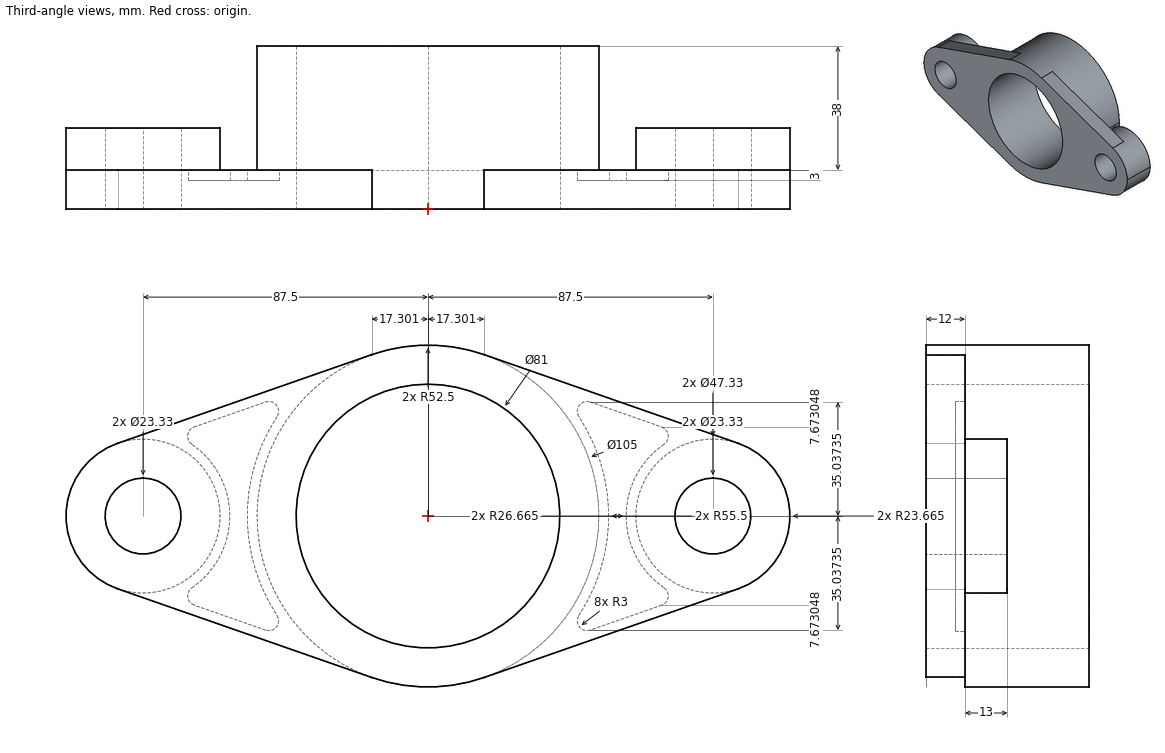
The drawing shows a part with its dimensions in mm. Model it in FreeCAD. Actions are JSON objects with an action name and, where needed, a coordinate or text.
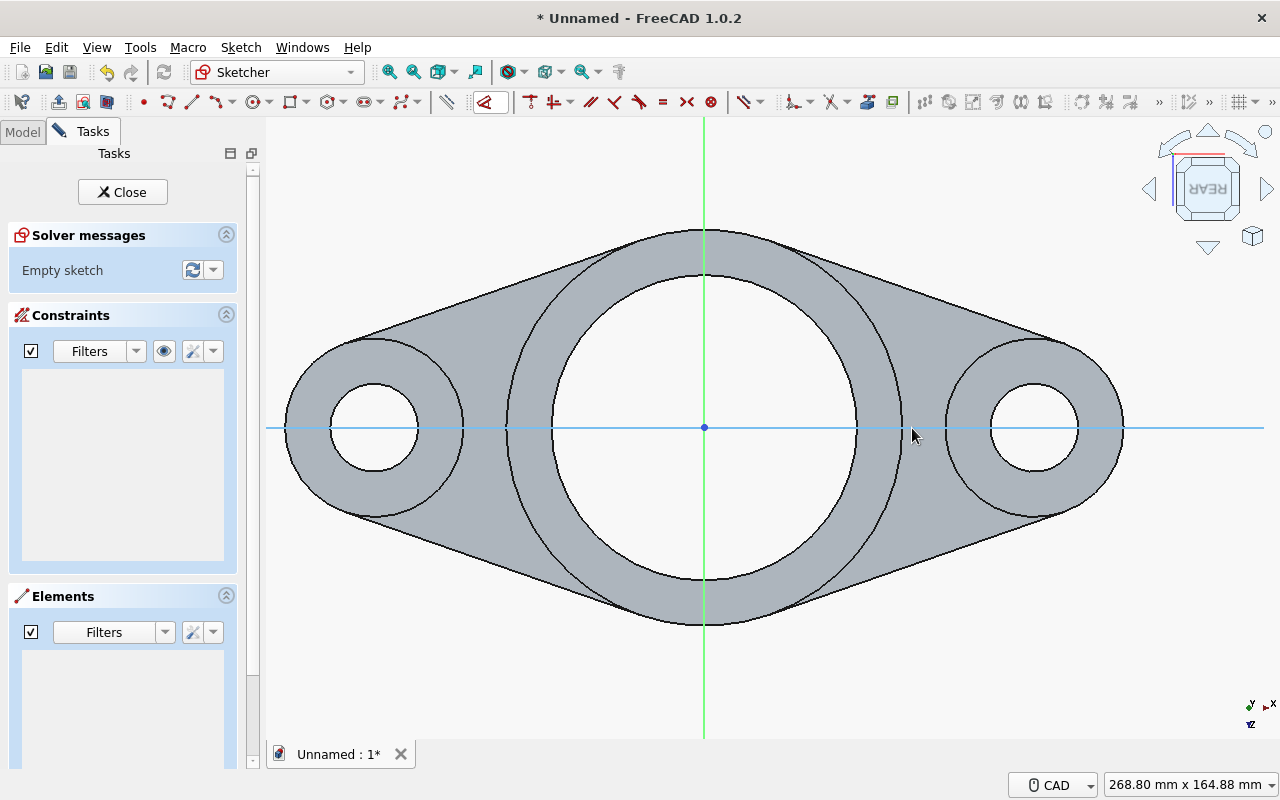
{"action": "left_click", "coordinate": [192, 102]}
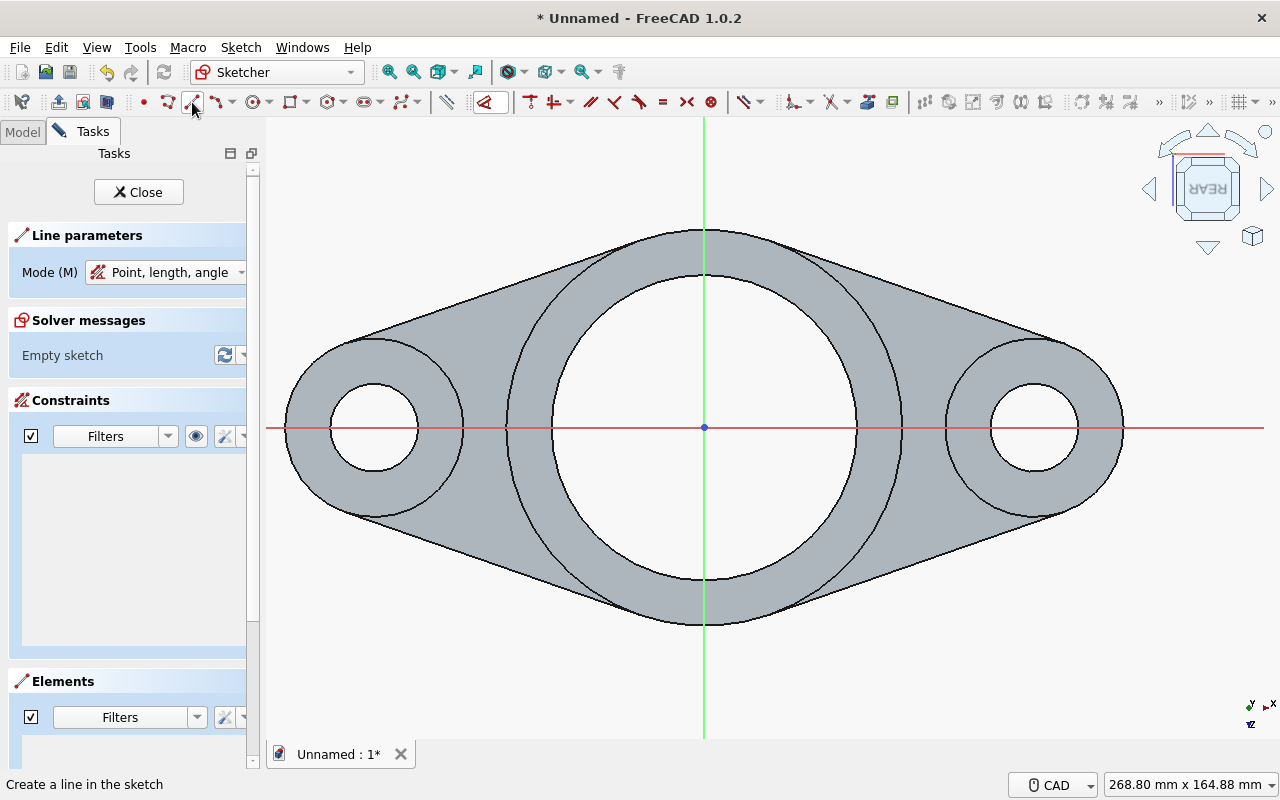
{"action": "left_click", "coordinate": [975, 325]}
{"action": "left_click", "coordinate": [892, 296]}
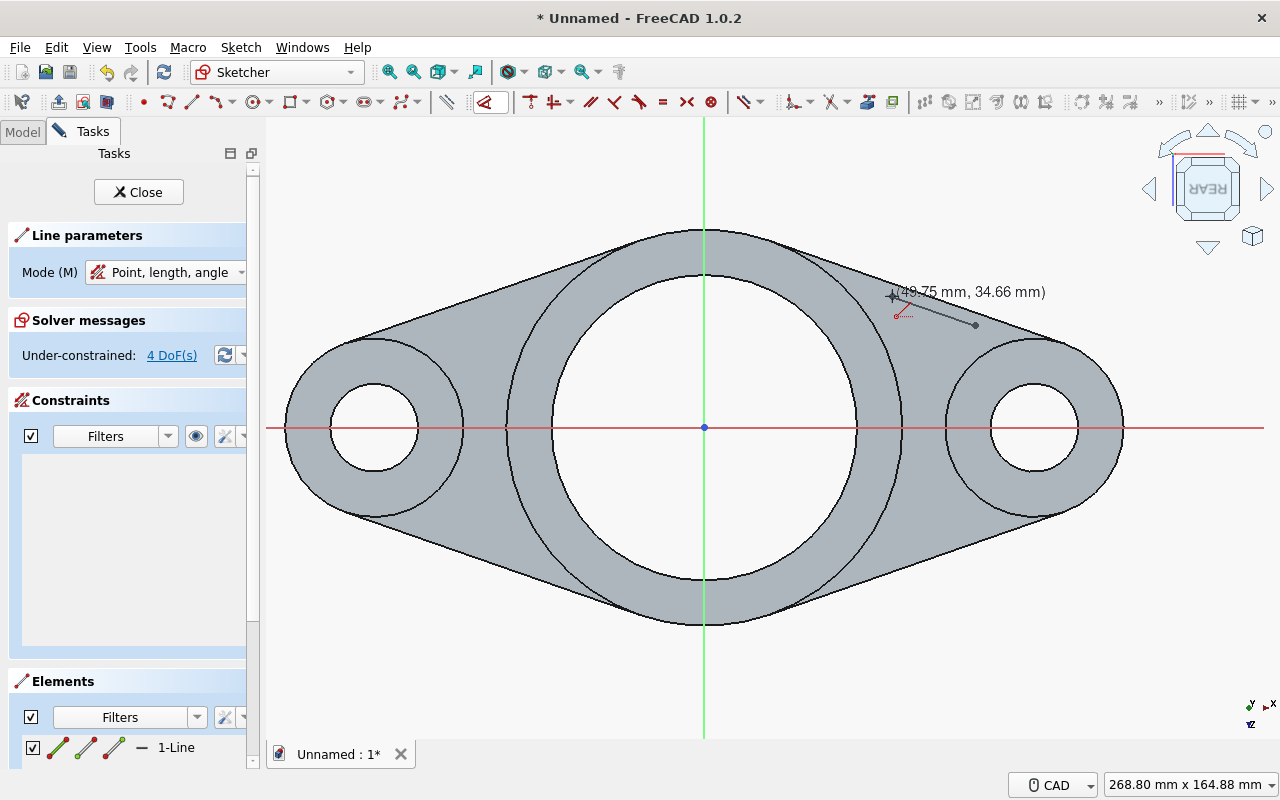
{"action": "left_click", "coordinate": [892, 560]}
{"action": "left_click", "coordinate": [975, 531]}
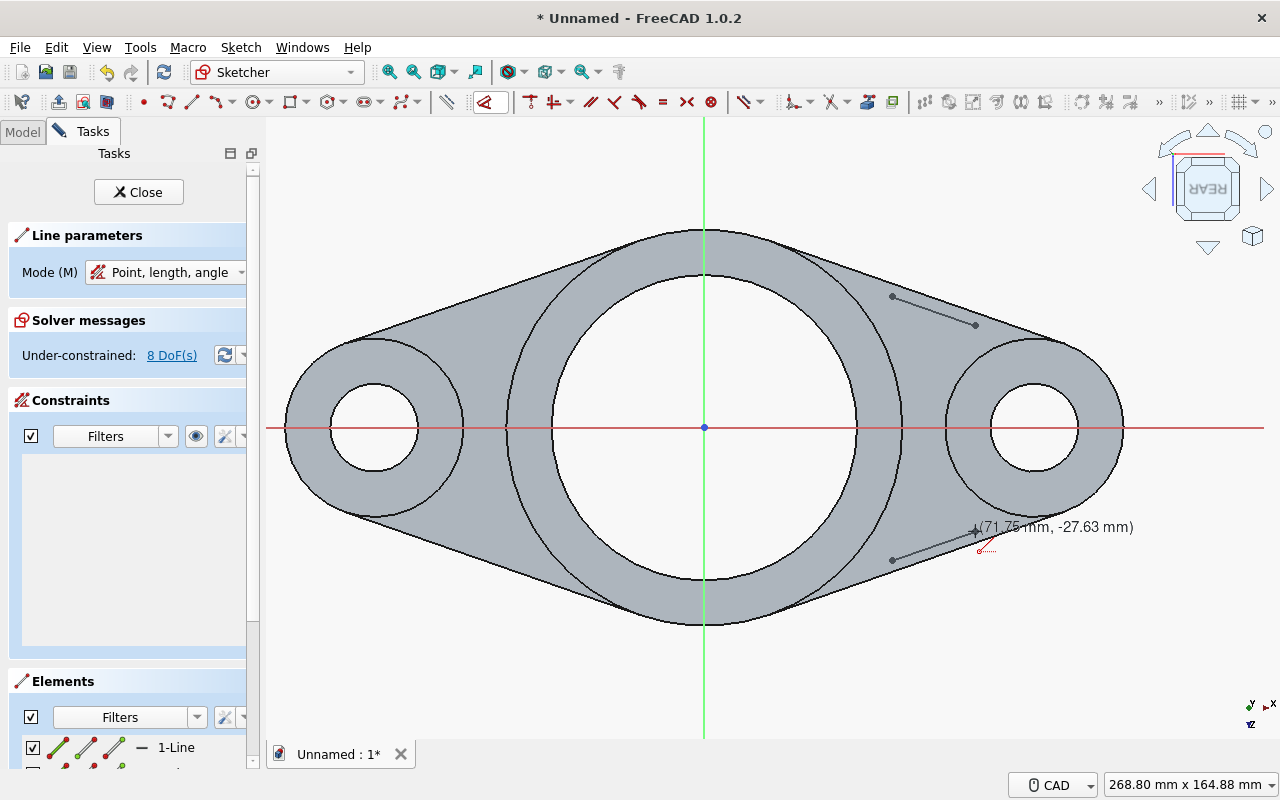
{"action": "left_click", "coordinate": [216, 102]}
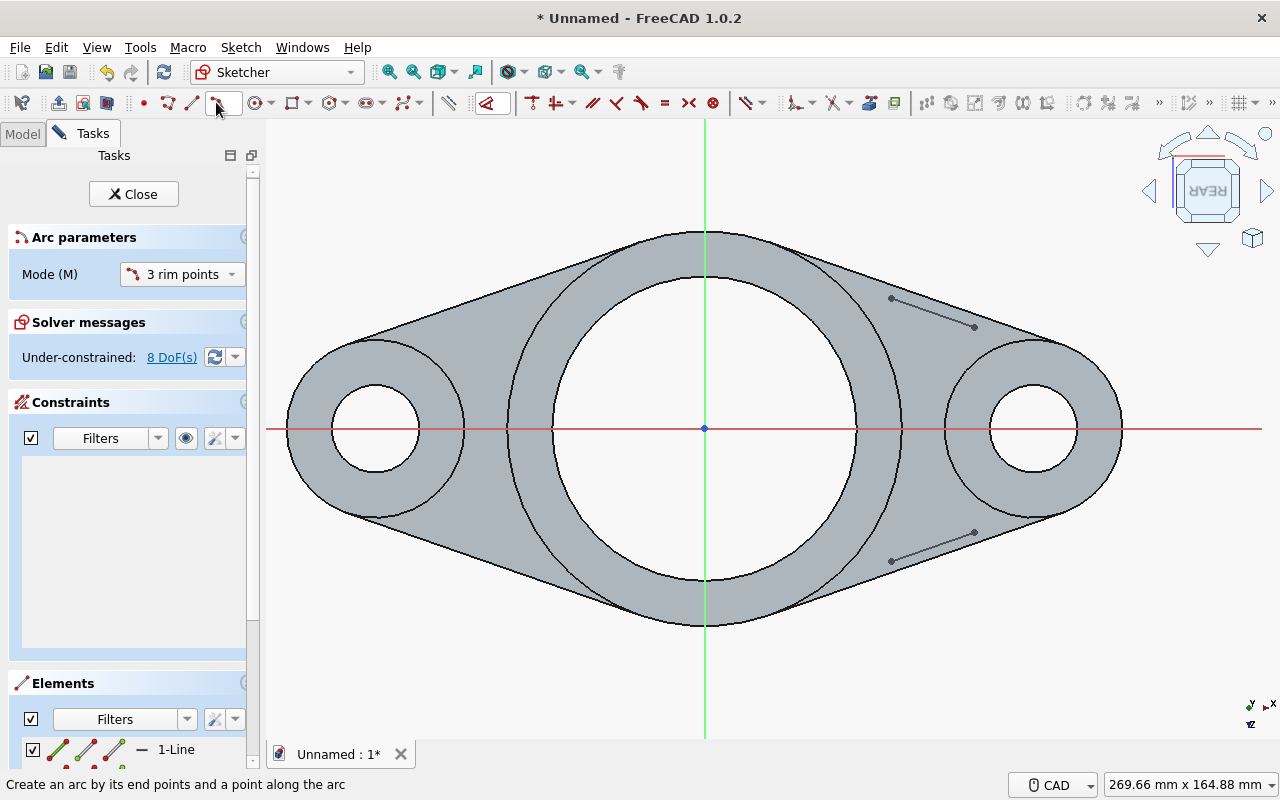
{"action": "left_click", "coordinate": [892, 298]}
{"action": "left_click", "coordinate": [879, 314]}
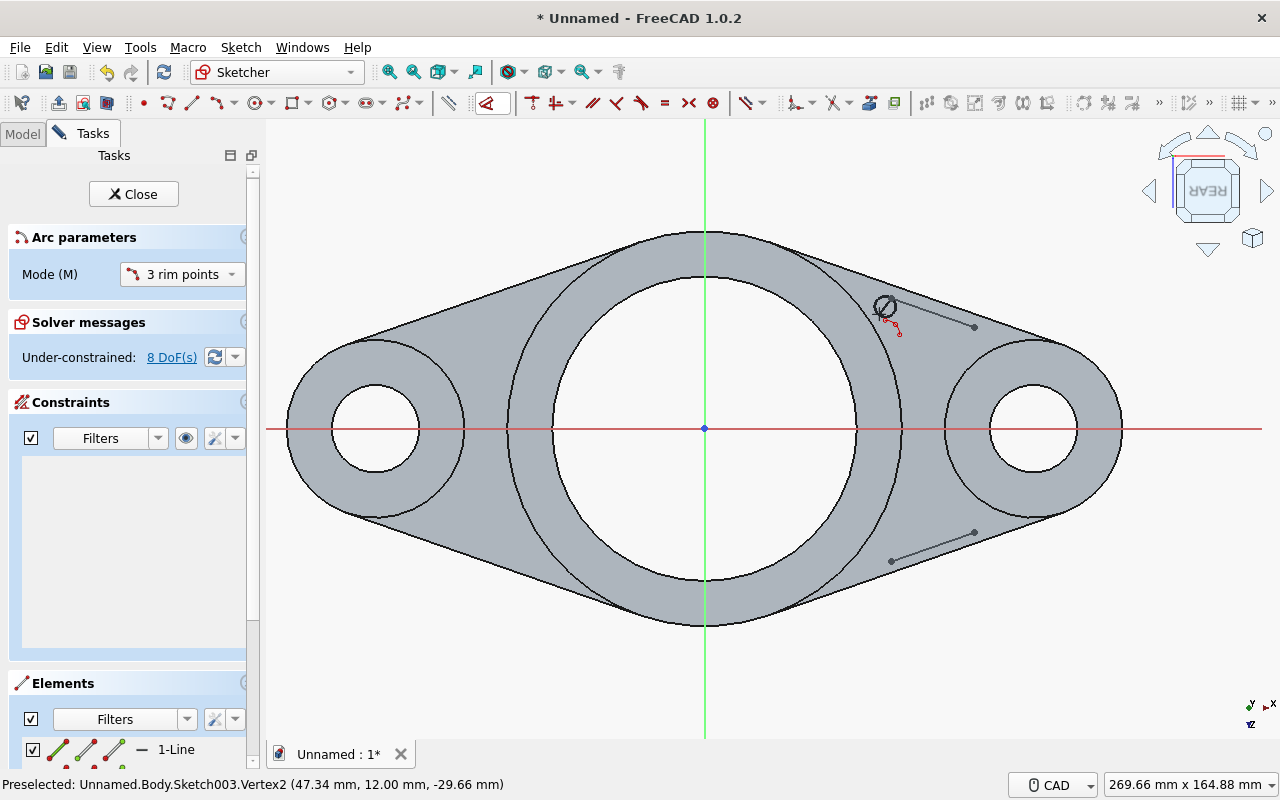
{"action": "scroll", "coordinate": [879, 301], "scroll_direction": "up", "scroll_amount": 4}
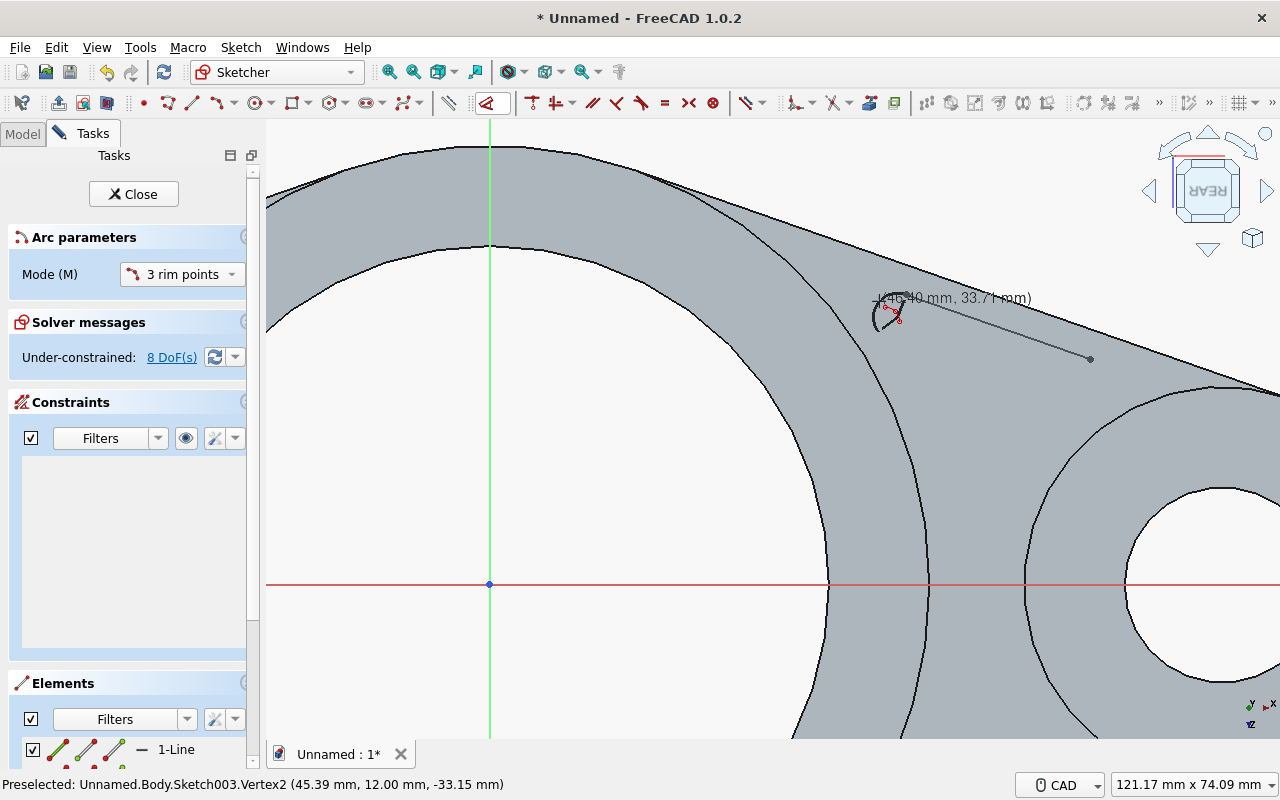
{"action": "left_click", "coordinate": [879, 300]}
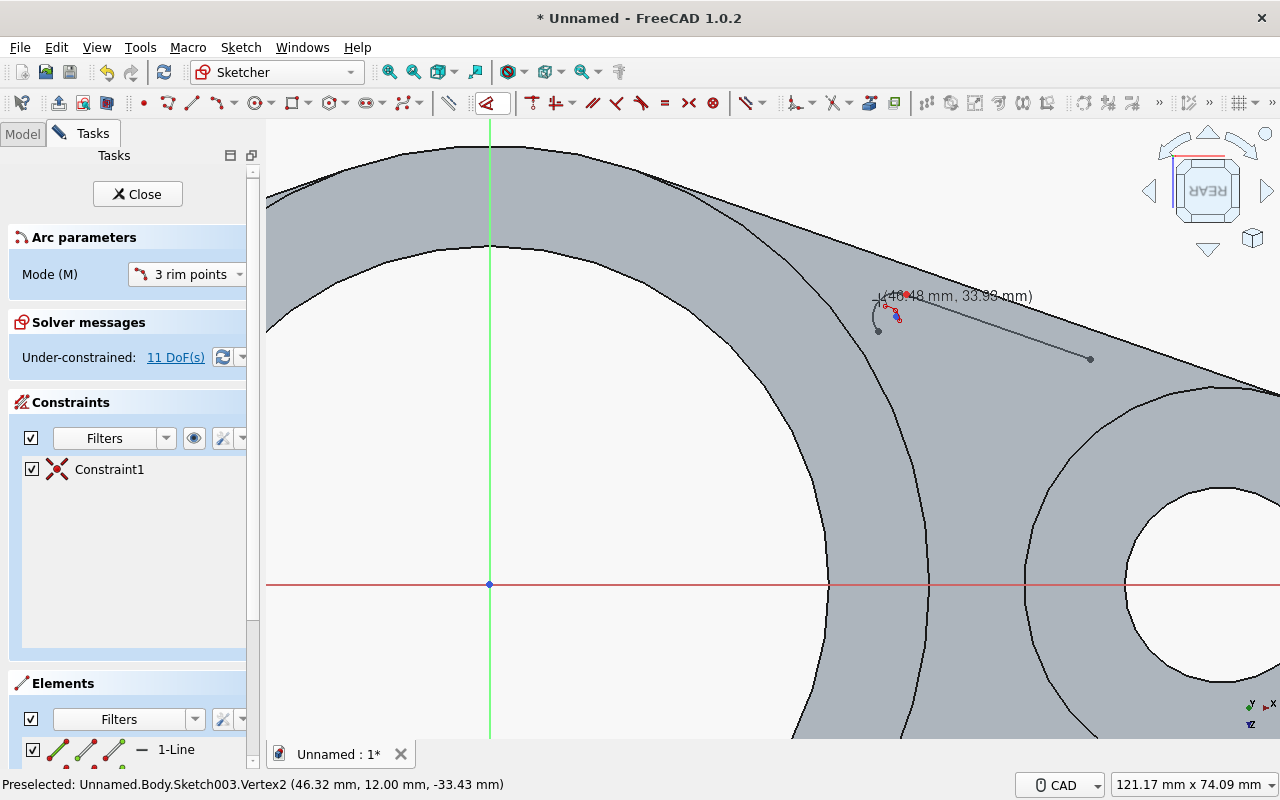
{"action": "left_click", "coordinate": [878, 332]}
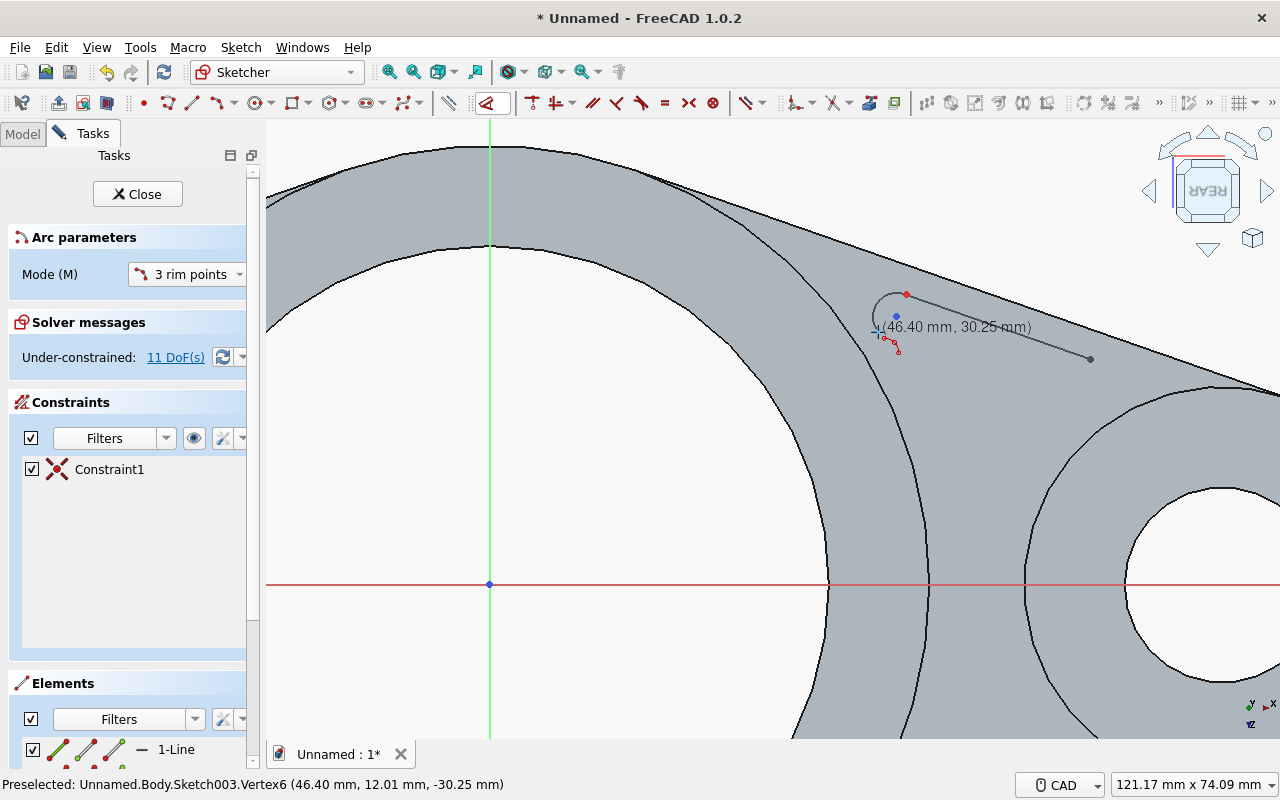
{"action": "scroll", "coordinate": [880, 302], "scroll_direction": "down", "scroll_amount": 4}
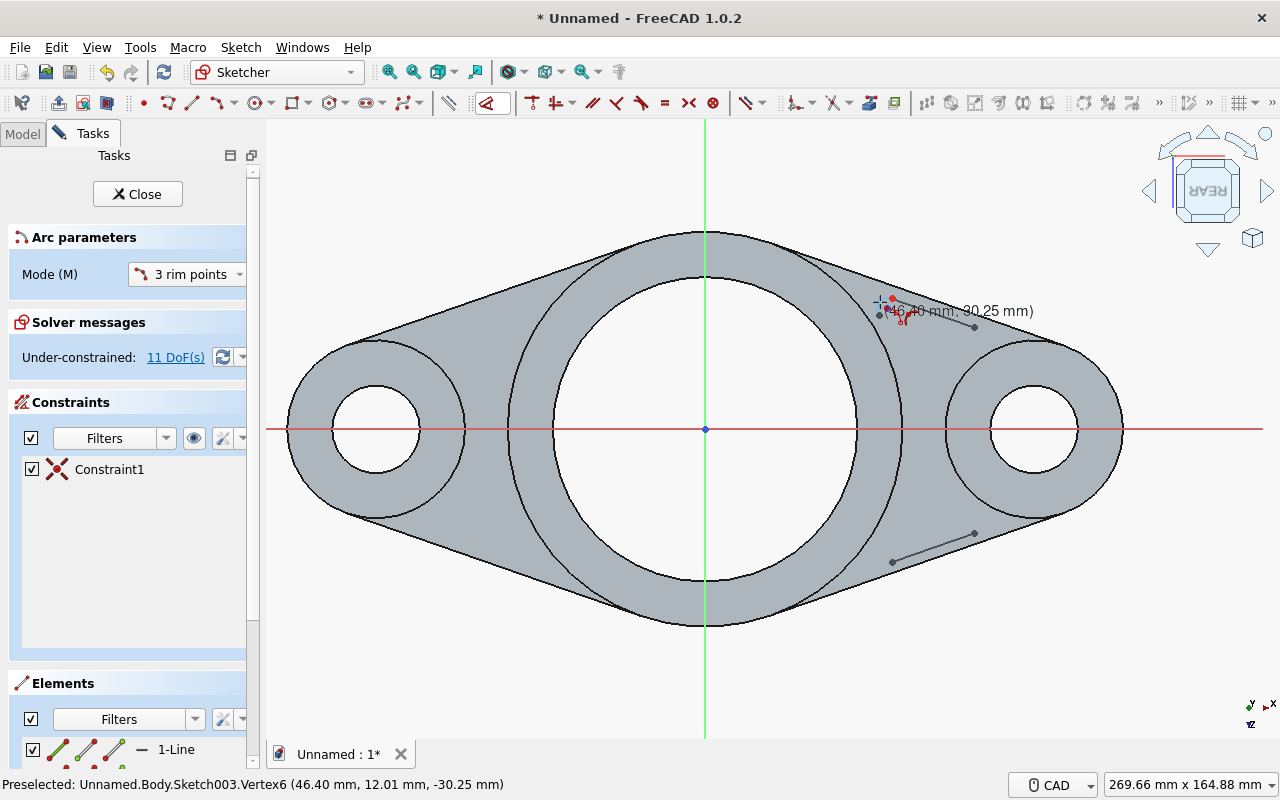
{"action": "left_click", "coordinate": [879, 544]}
{"action": "left_click", "coordinate": [912, 454]}